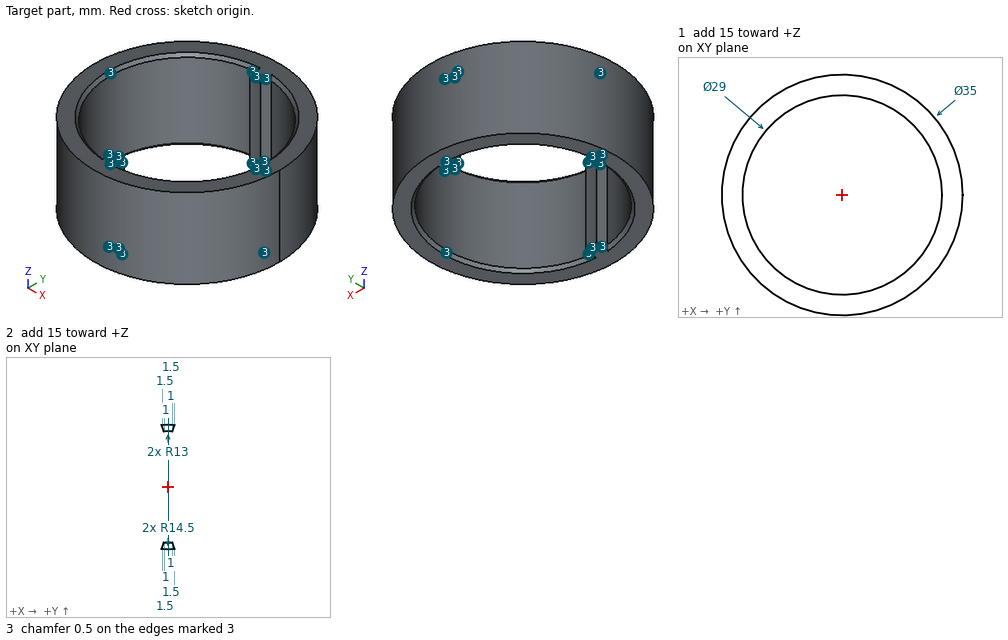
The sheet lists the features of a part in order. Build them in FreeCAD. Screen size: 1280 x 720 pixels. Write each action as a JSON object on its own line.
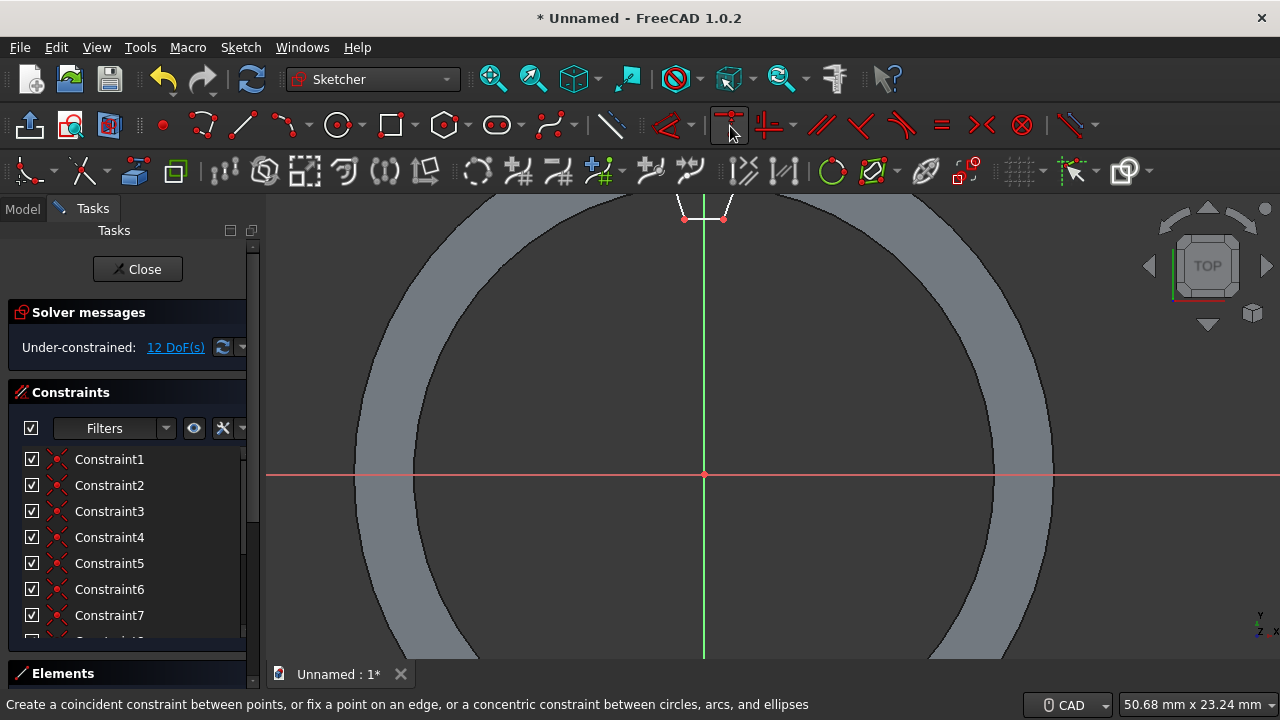
{"action": "scroll", "coordinate": [705, 368], "scroll_direction": "down", "scroll_amount": 3}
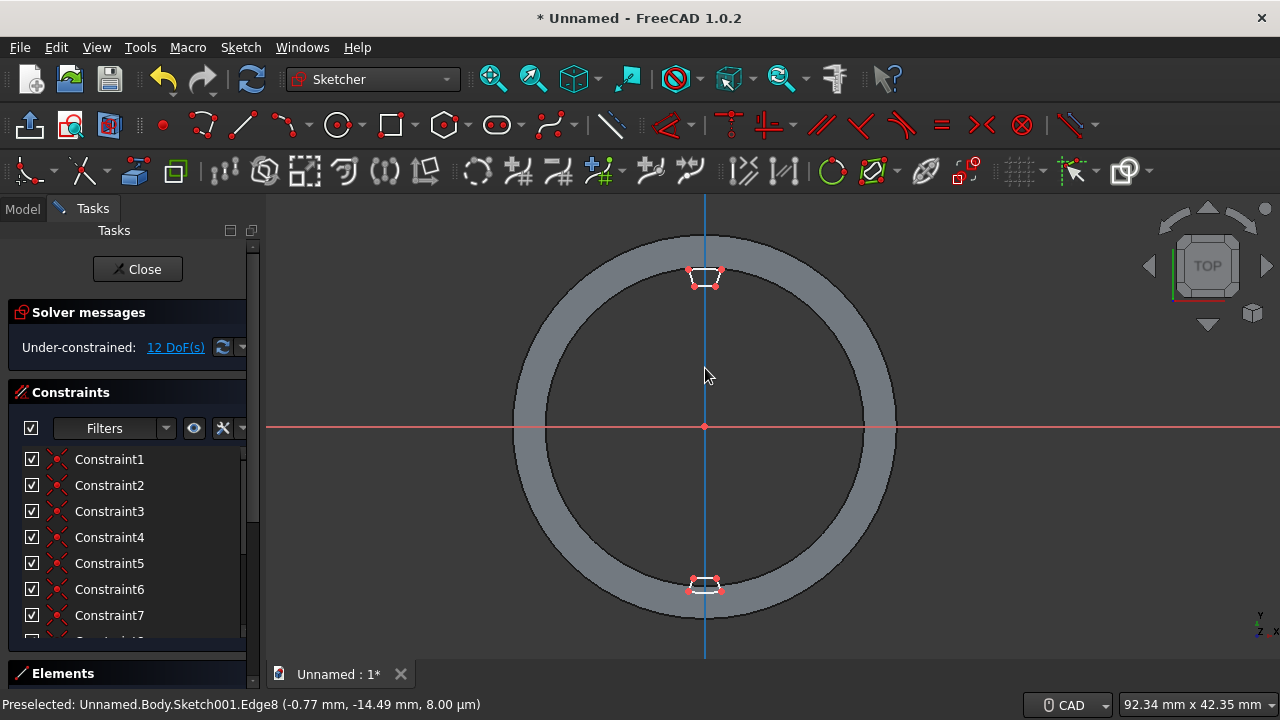
{"action": "scroll", "coordinate": [705, 286], "scroll_direction": "up", "scroll_amount": 2}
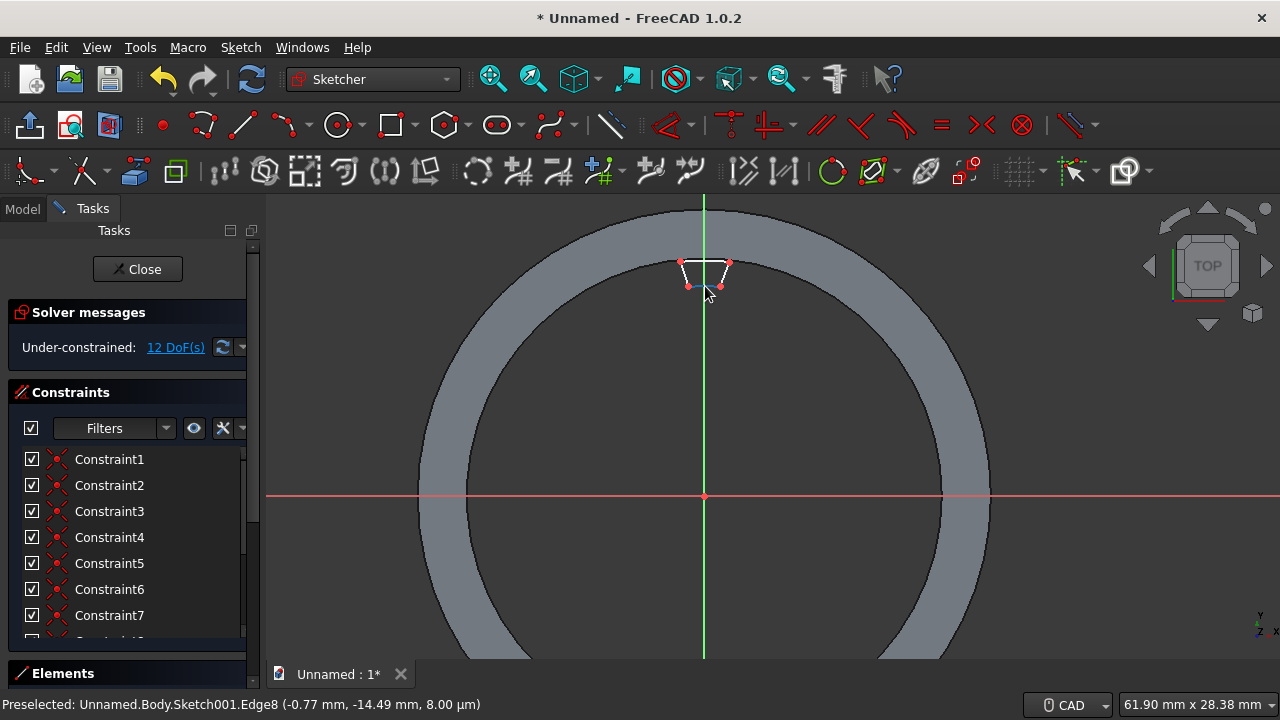
{"action": "left_click", "coordinate": [704, 286]}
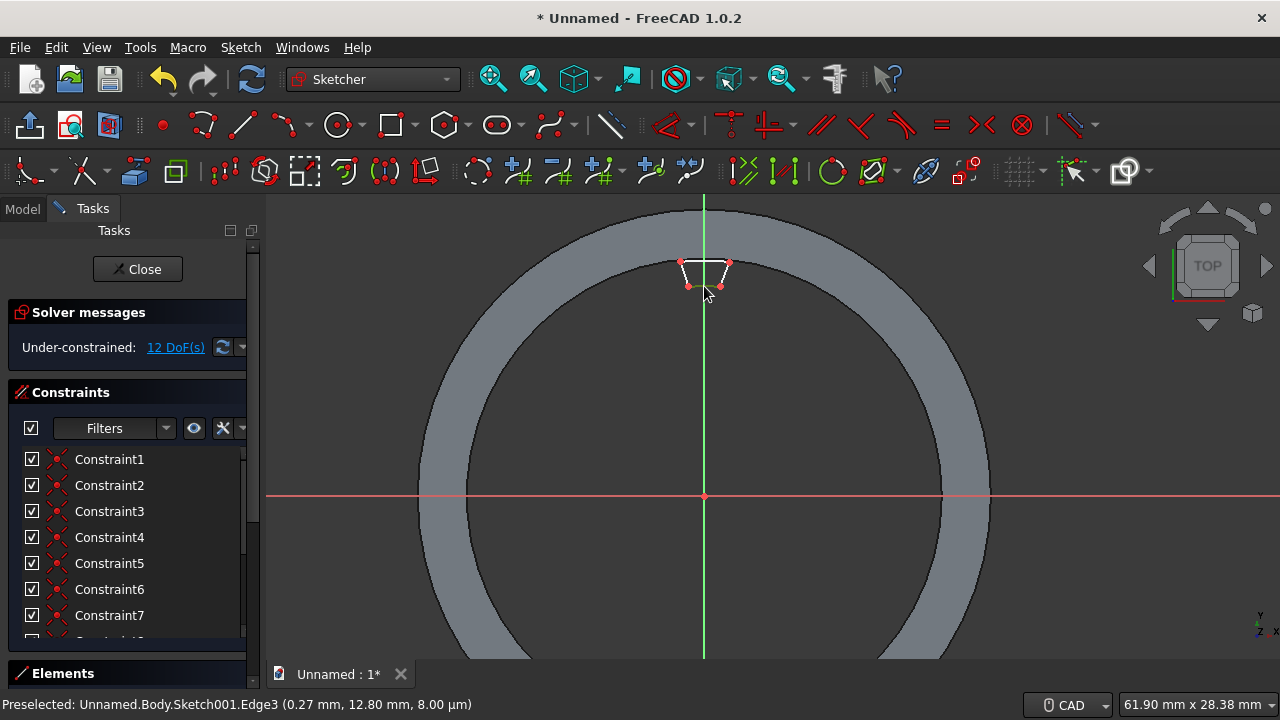
{"action": "scroll", "coordinate": [705, 285], "scroll_direction": "down", "scroll_amount": 2}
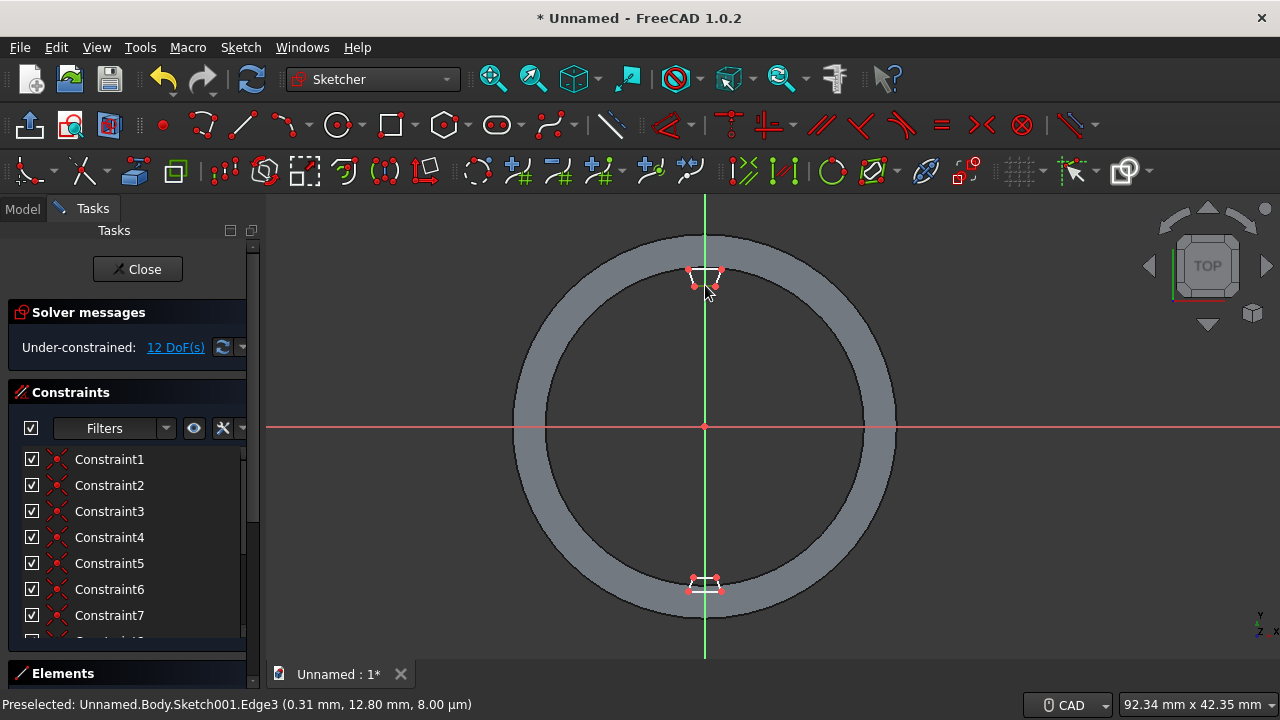
{"action": "left_click", "coordinate": [705, 578]}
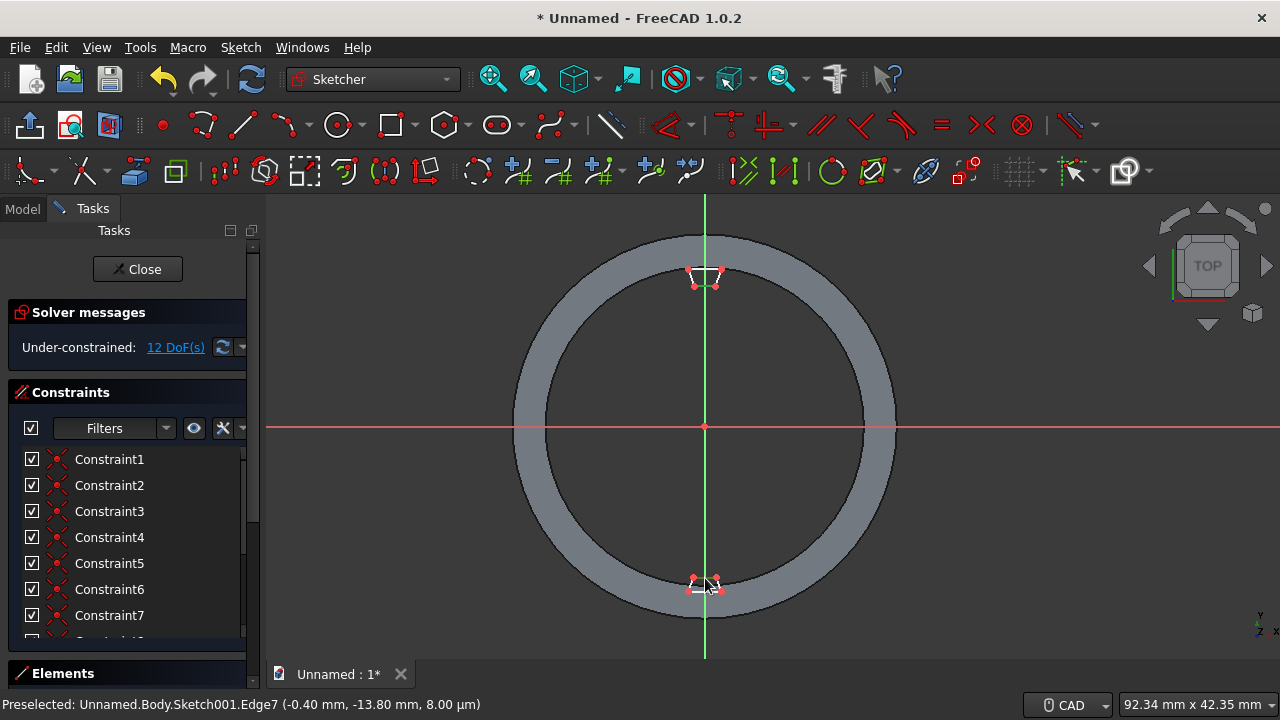
{"action": "left_click", "coordinate": [942, 126]}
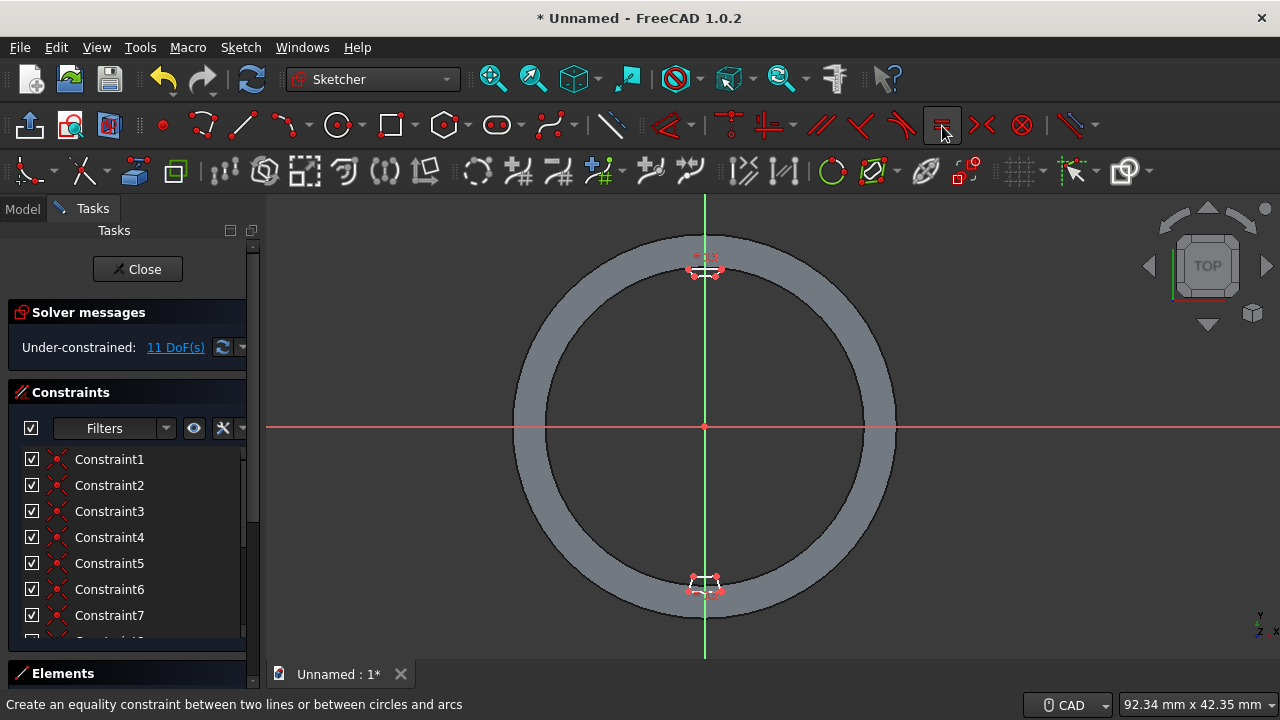
{"action": "scroll", "coordinate": [705, 269], "scroll_direction": "up", "scroll_amount": 4}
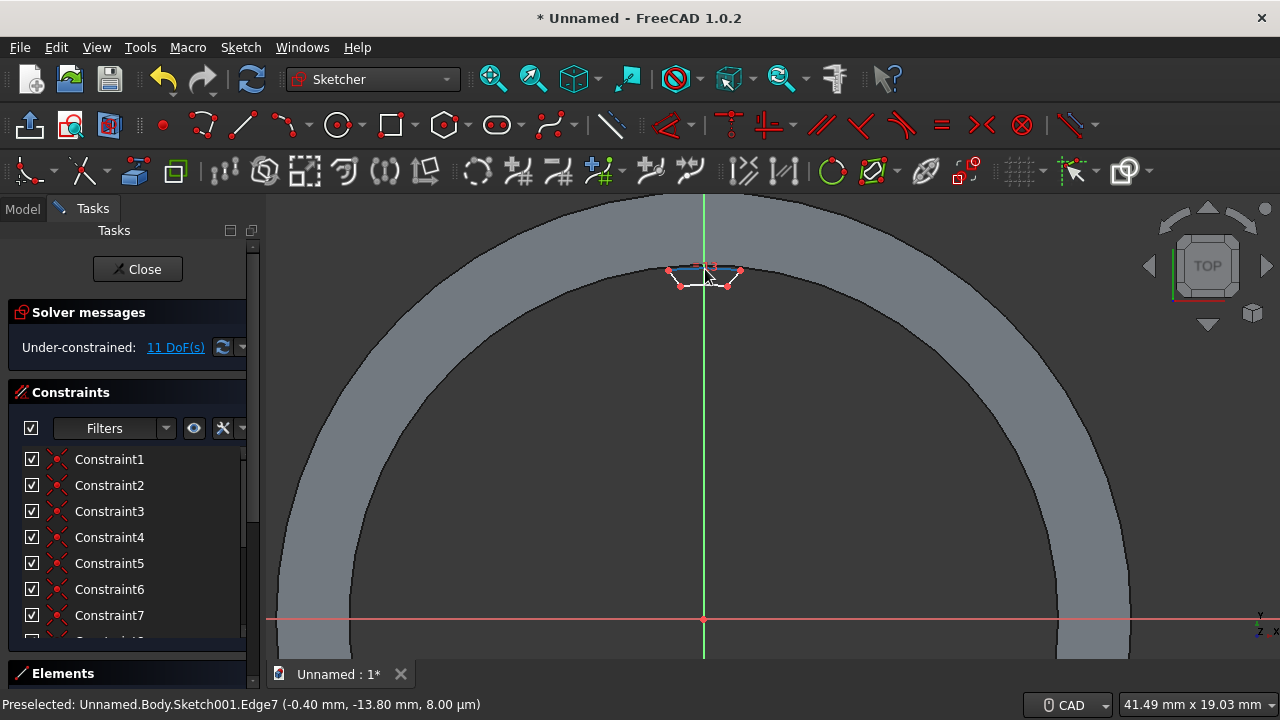
{"action": "left_click", "coordinate": [719, 269]}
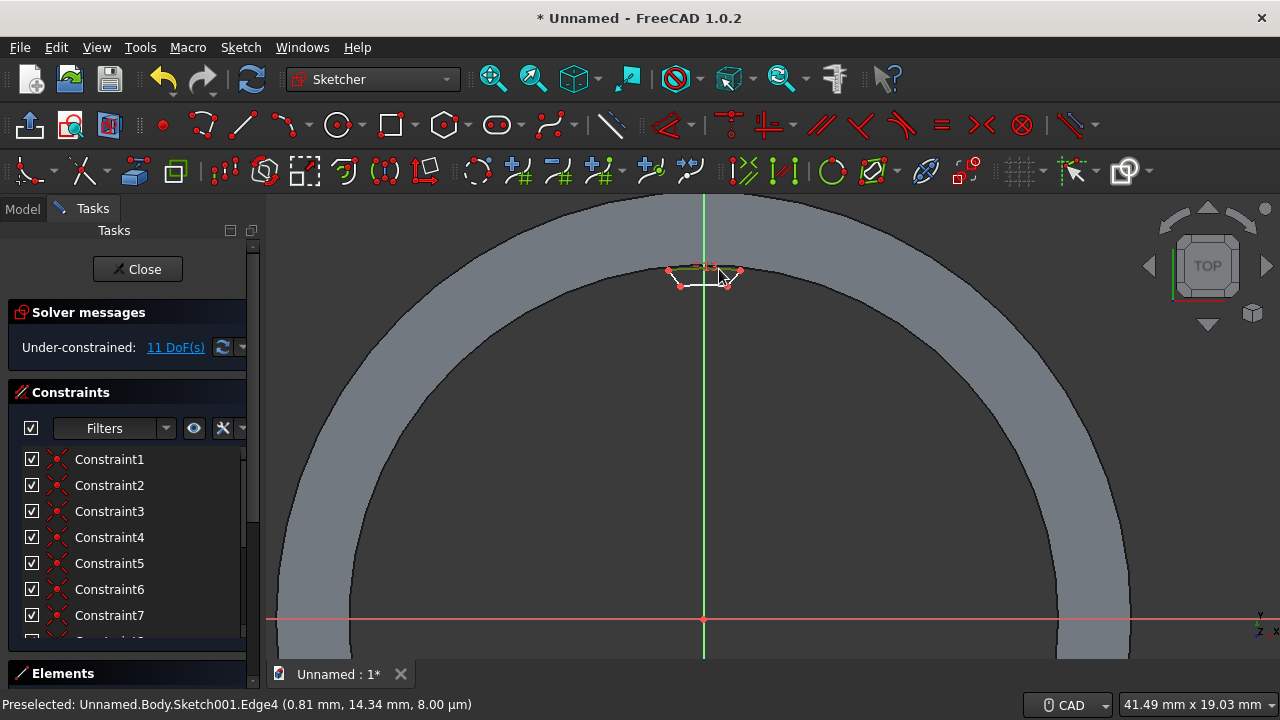
{"action": "scroll", "coordinate": [705, 269], "scroll_direction": "down", "scroll_amount": 4}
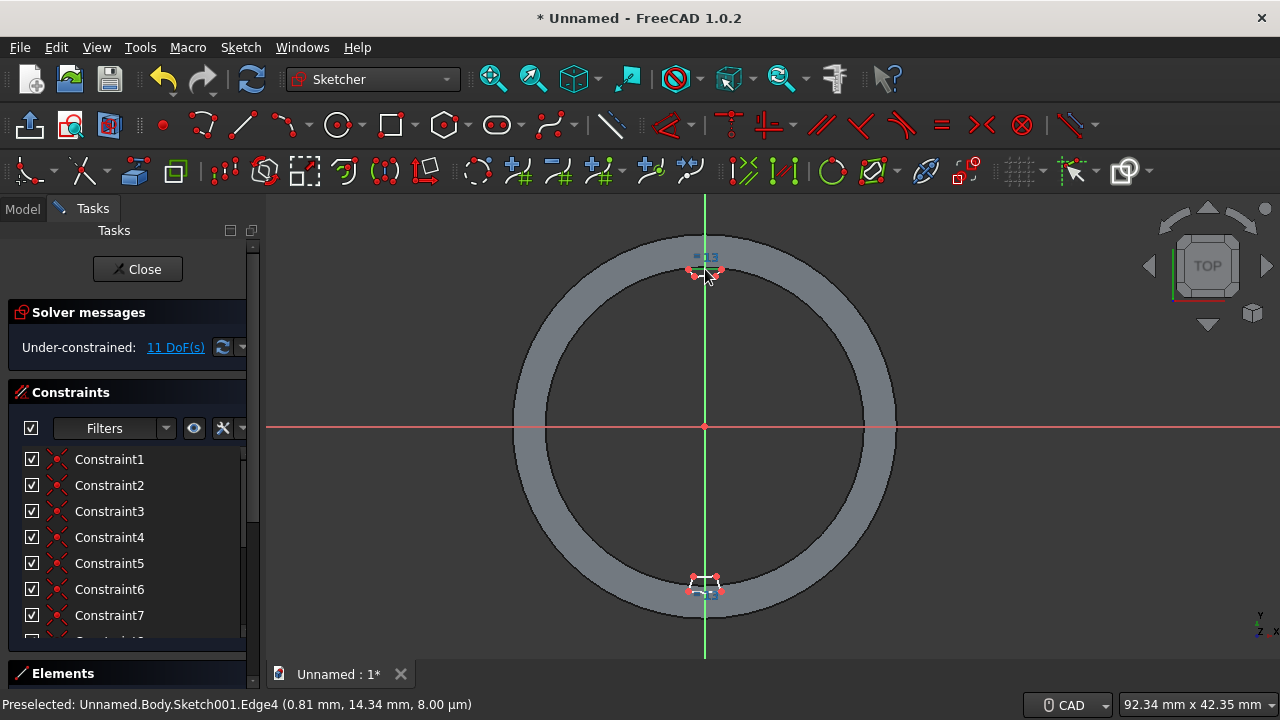
{"action": "scroll", "coordinate": [698, 592], "scroll_direction": "up", "scroll_amount": 4}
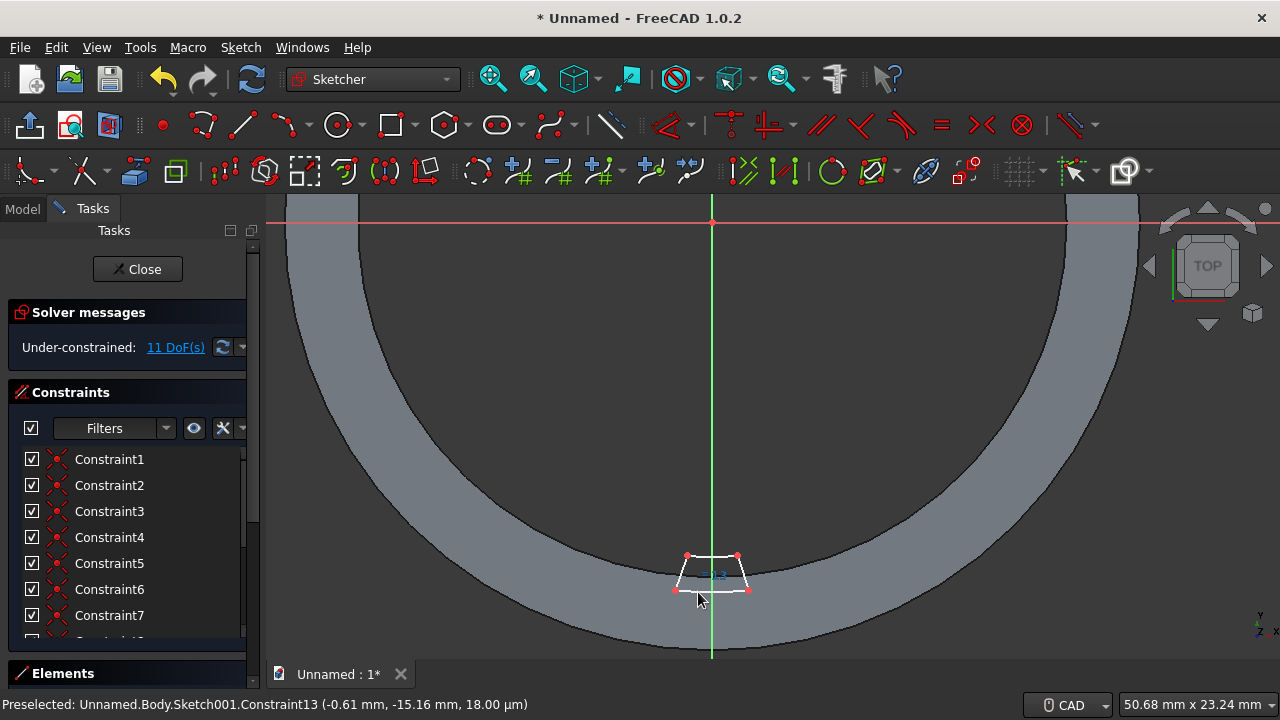
{"action": "left_click", "coordinate": [697, 592]}